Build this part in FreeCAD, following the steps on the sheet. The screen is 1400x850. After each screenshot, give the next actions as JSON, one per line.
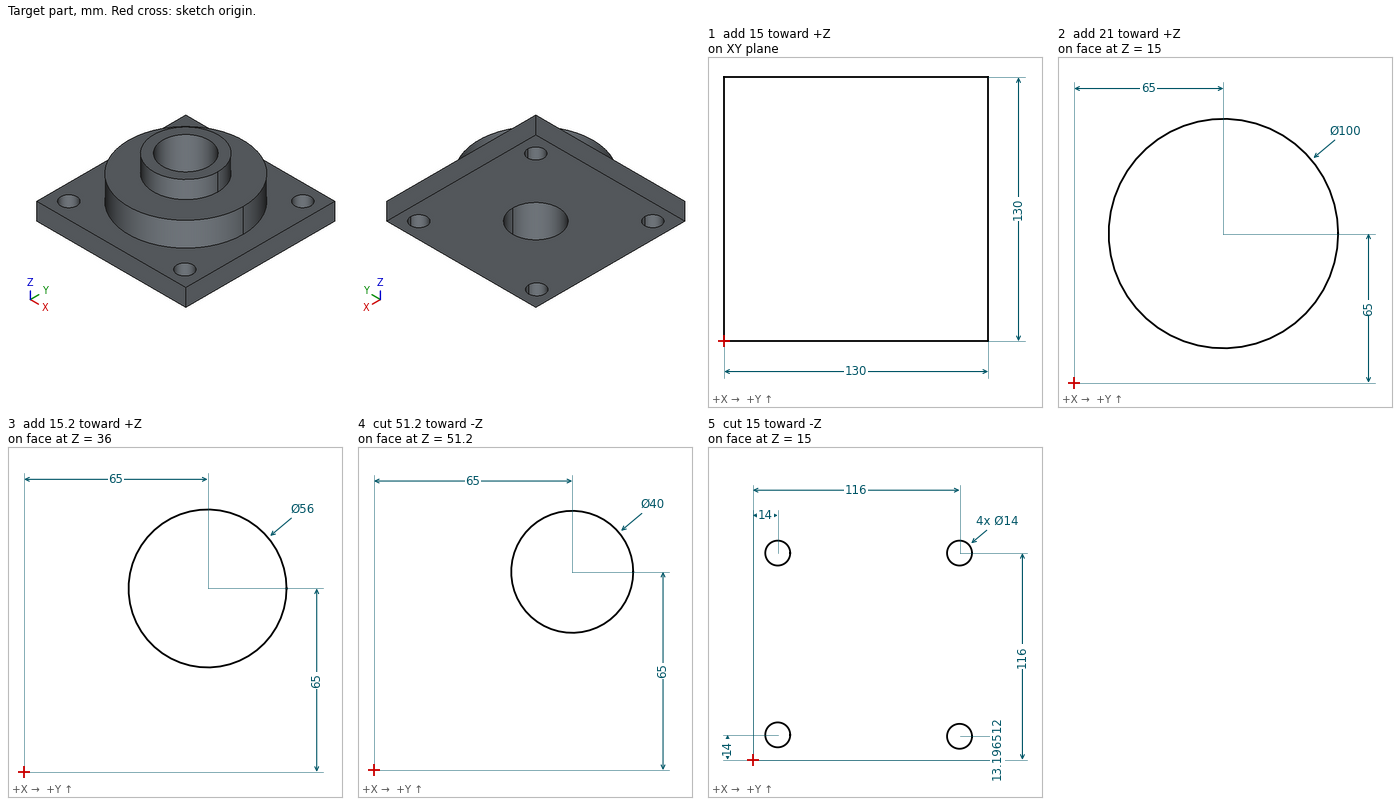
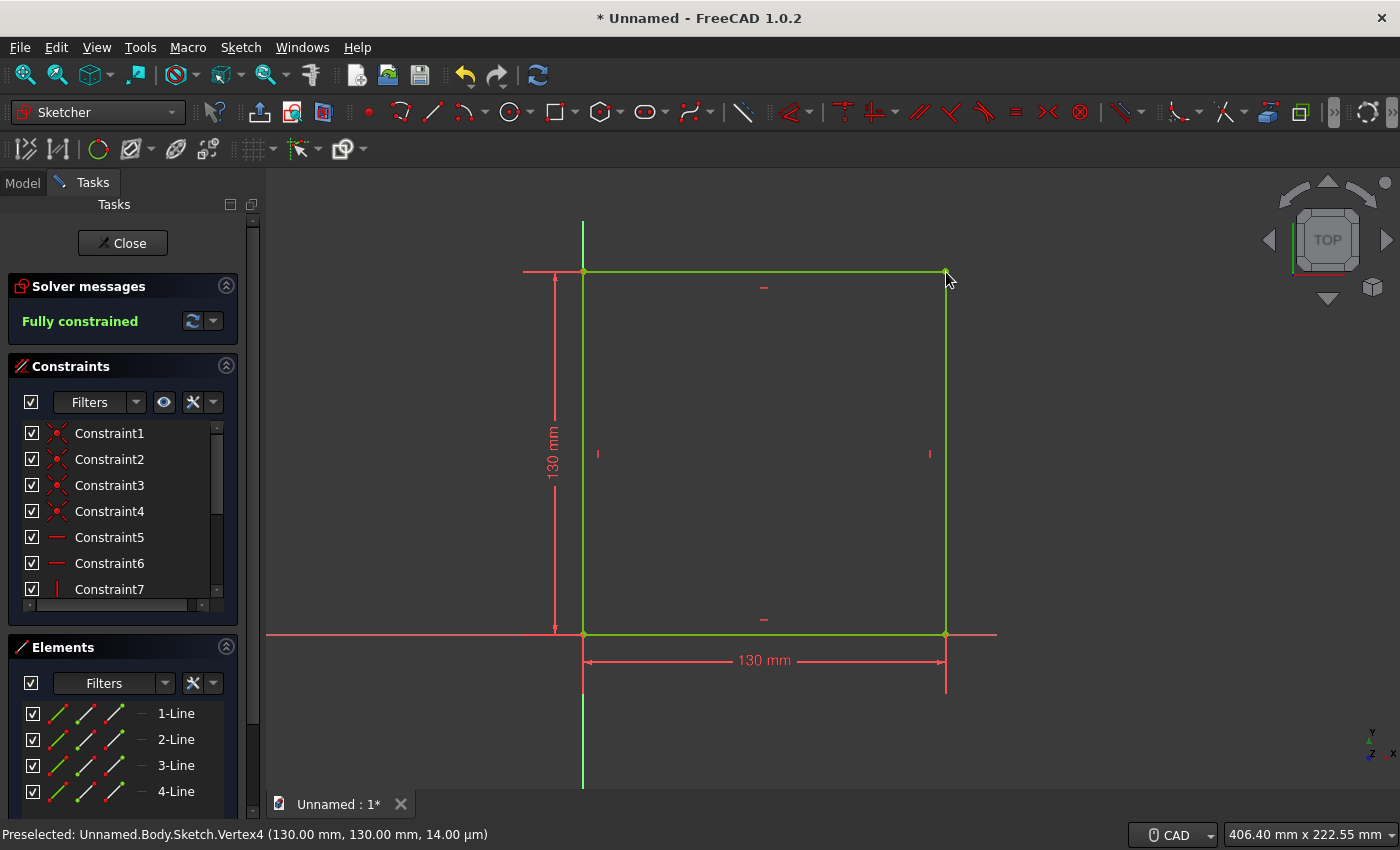
{"action": "left_click", "coordinate": [123, 243]}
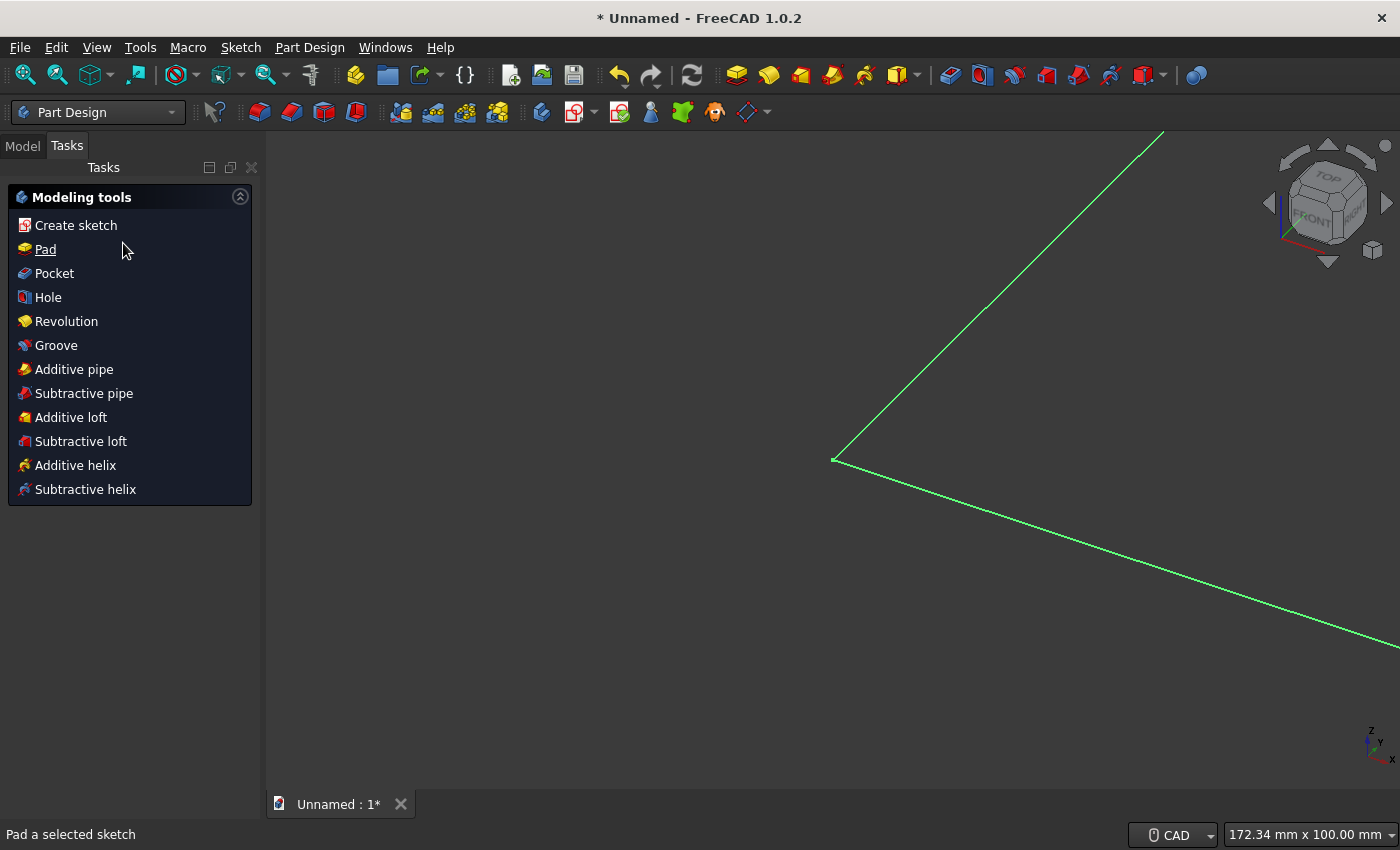
{"action": "left_click", "coordinate": [738, 76]}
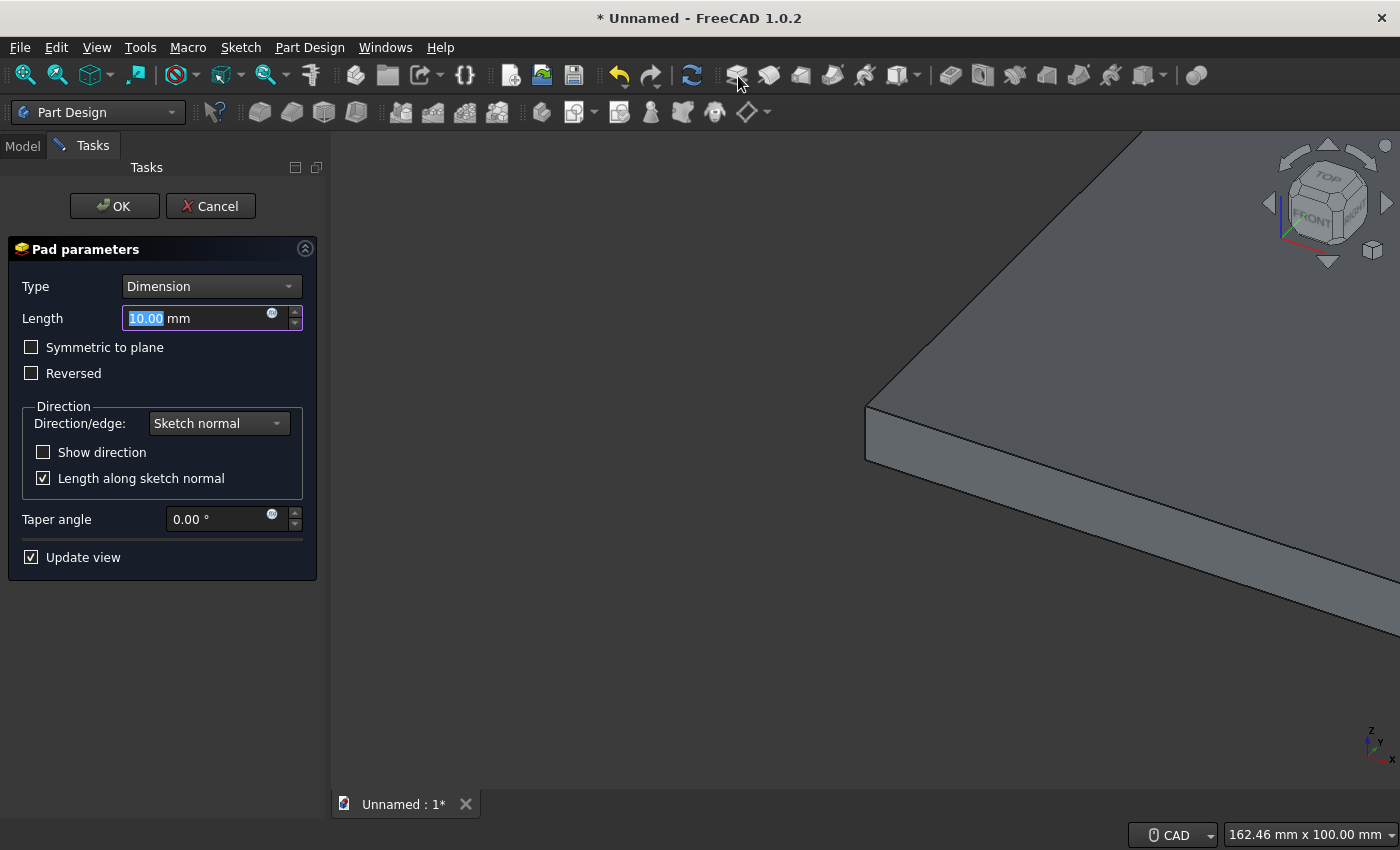
{"action": "type", "text": "15"}
{"action": "key", "text": "Tab"}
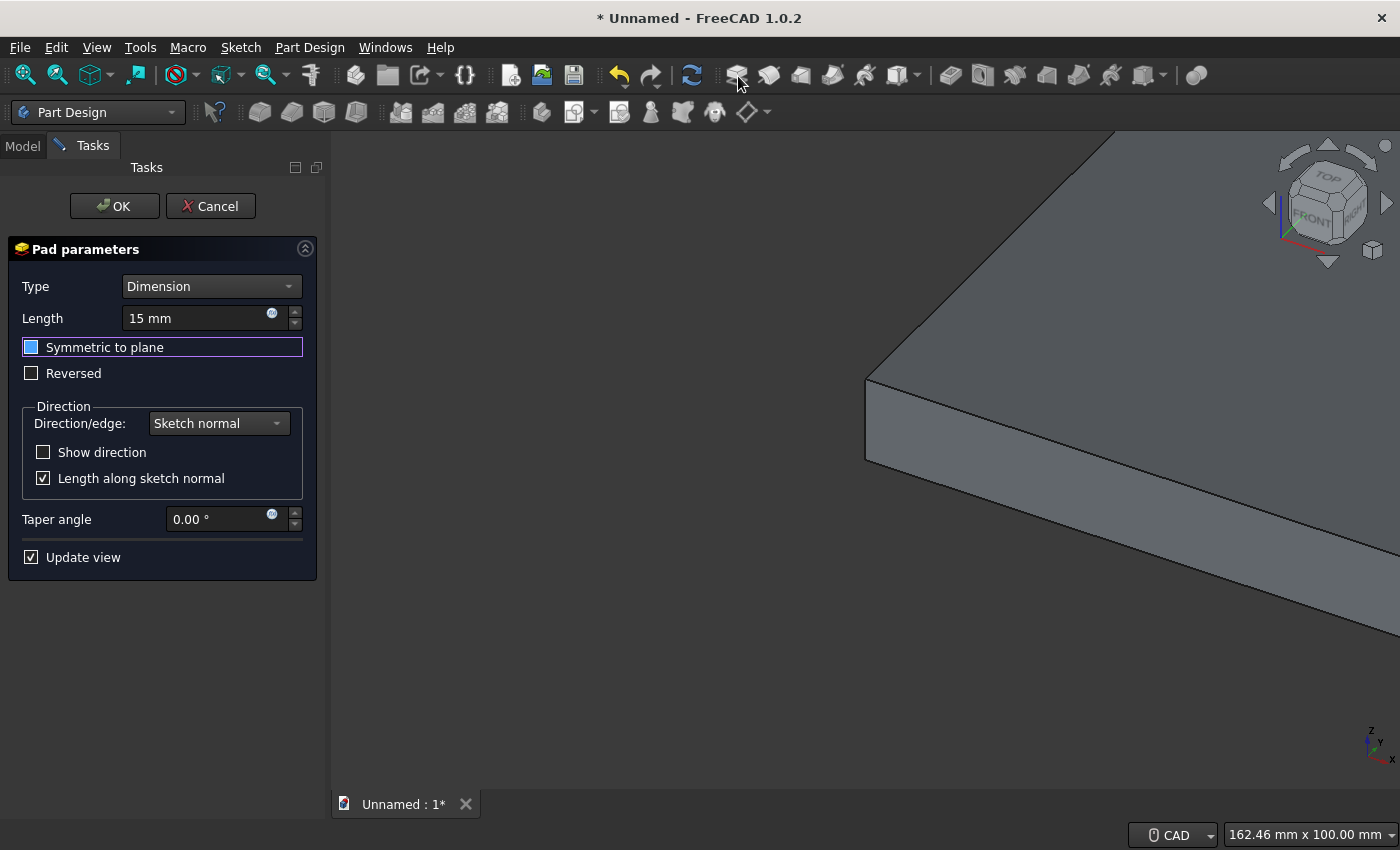
{"action": "left_click", "coordinate": [115, 206]}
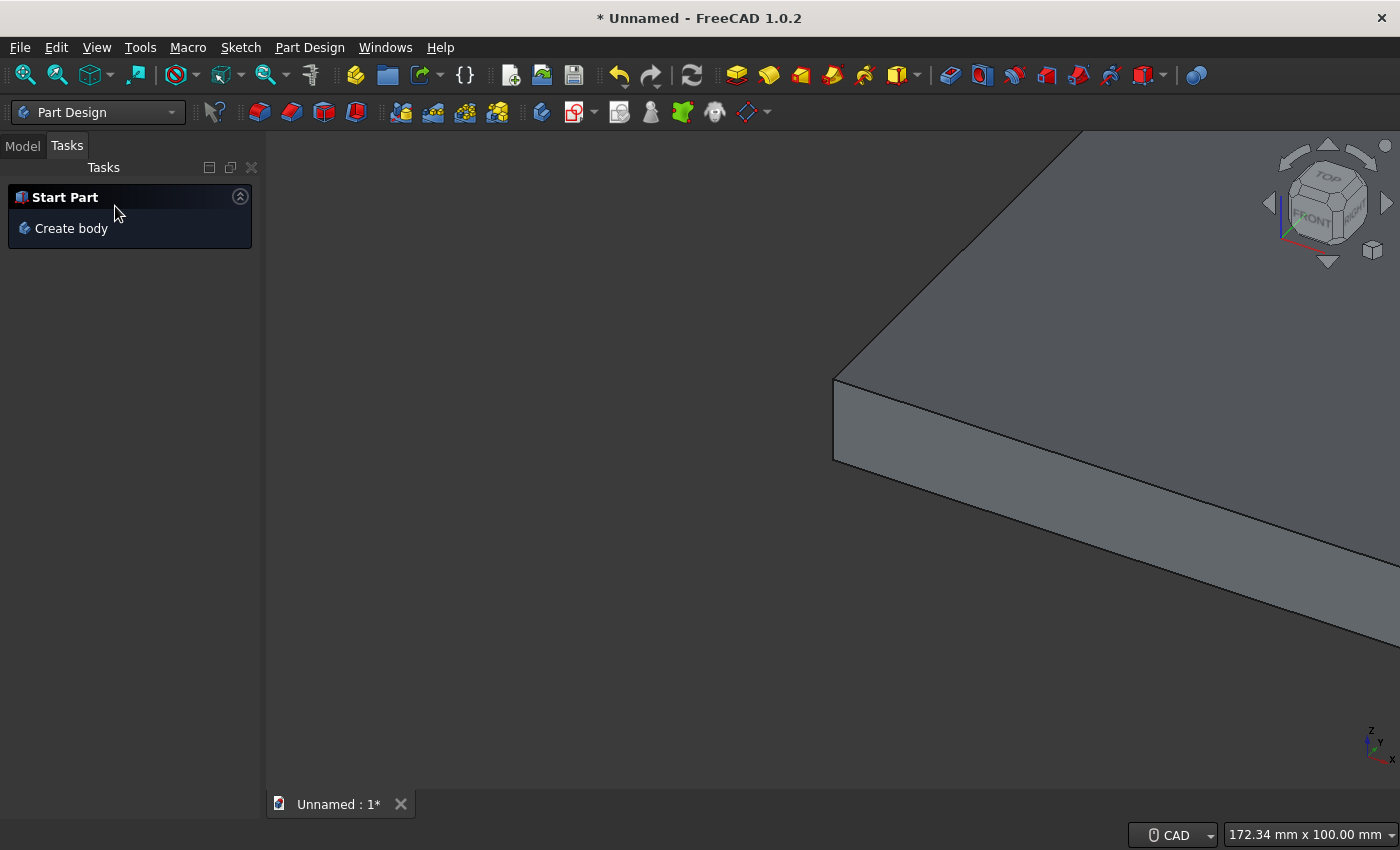
{"action": "key", "text": "v f"}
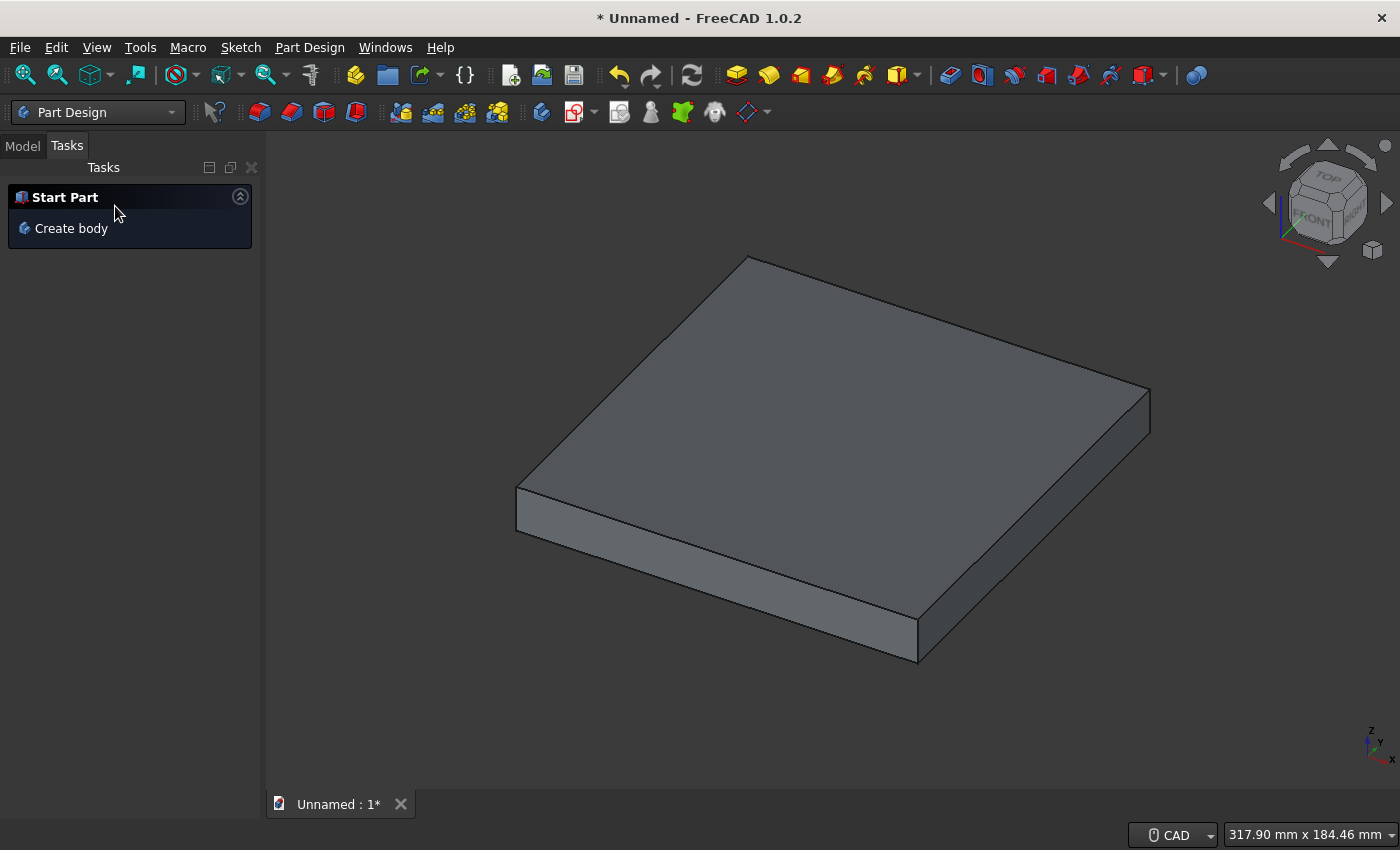
{"action": "left_click", "coordinate": [833, 437]}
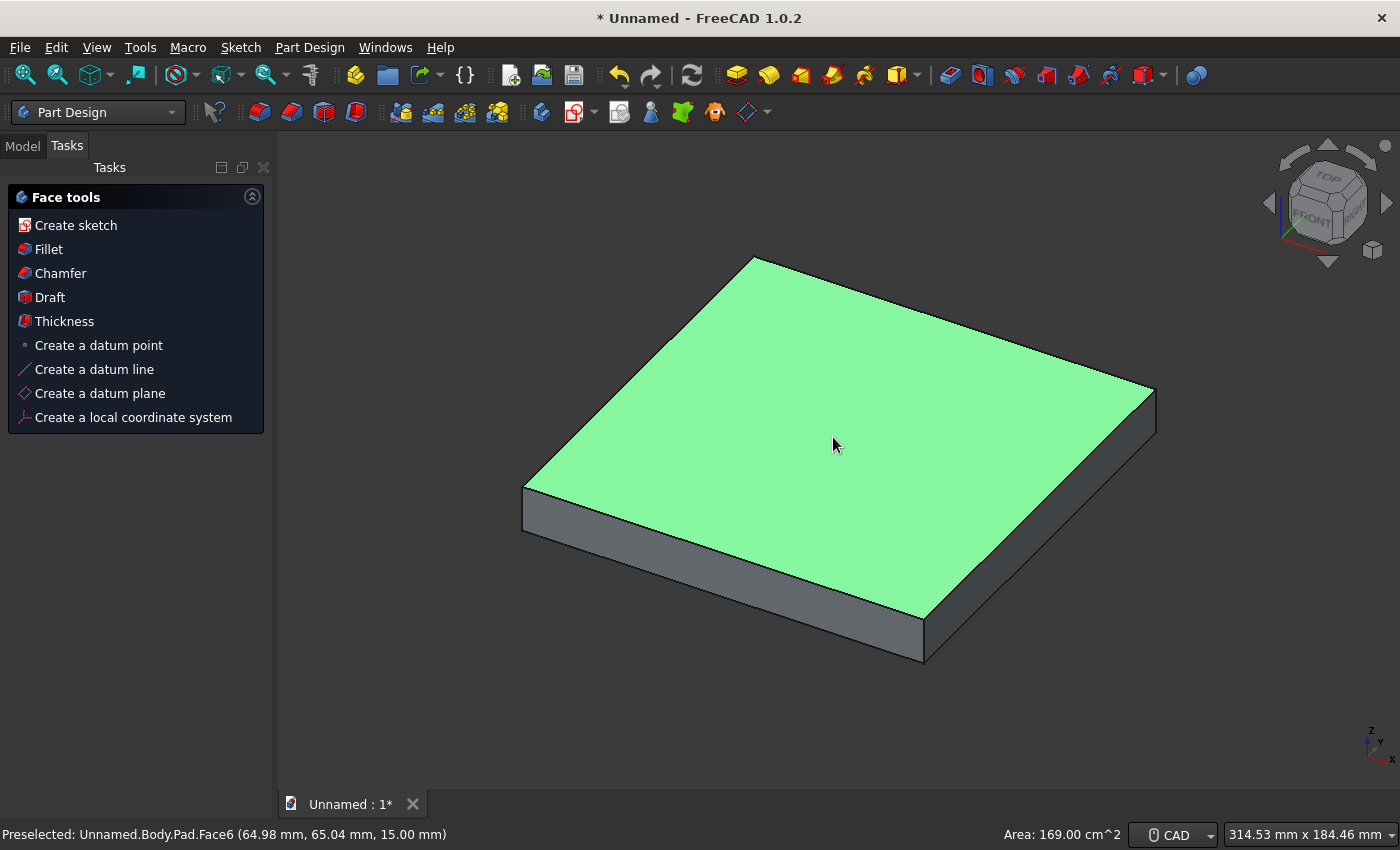
{"action": "left_click", "coordinate": [574, 112]}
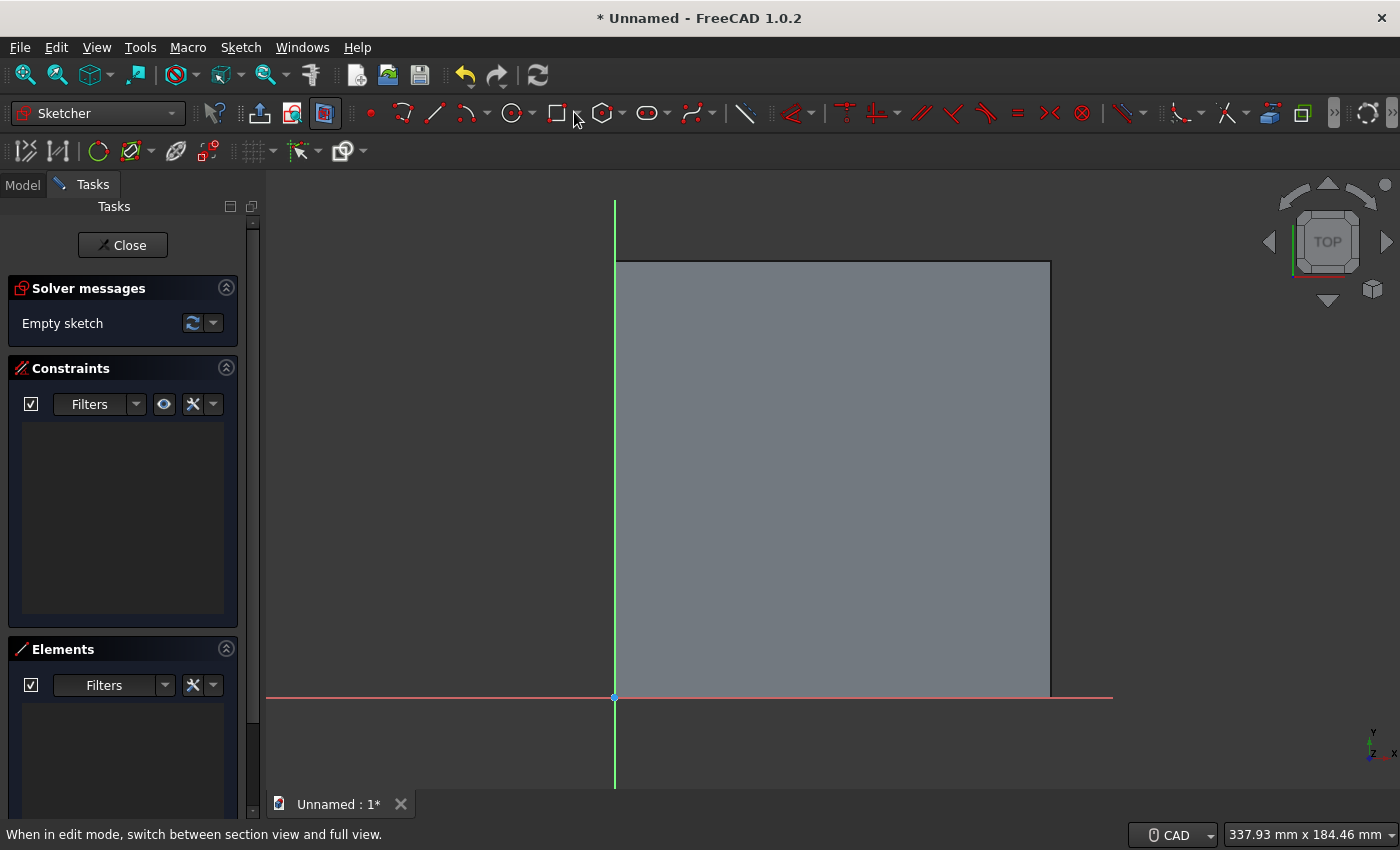
{"action": "key", "text": "g c"}